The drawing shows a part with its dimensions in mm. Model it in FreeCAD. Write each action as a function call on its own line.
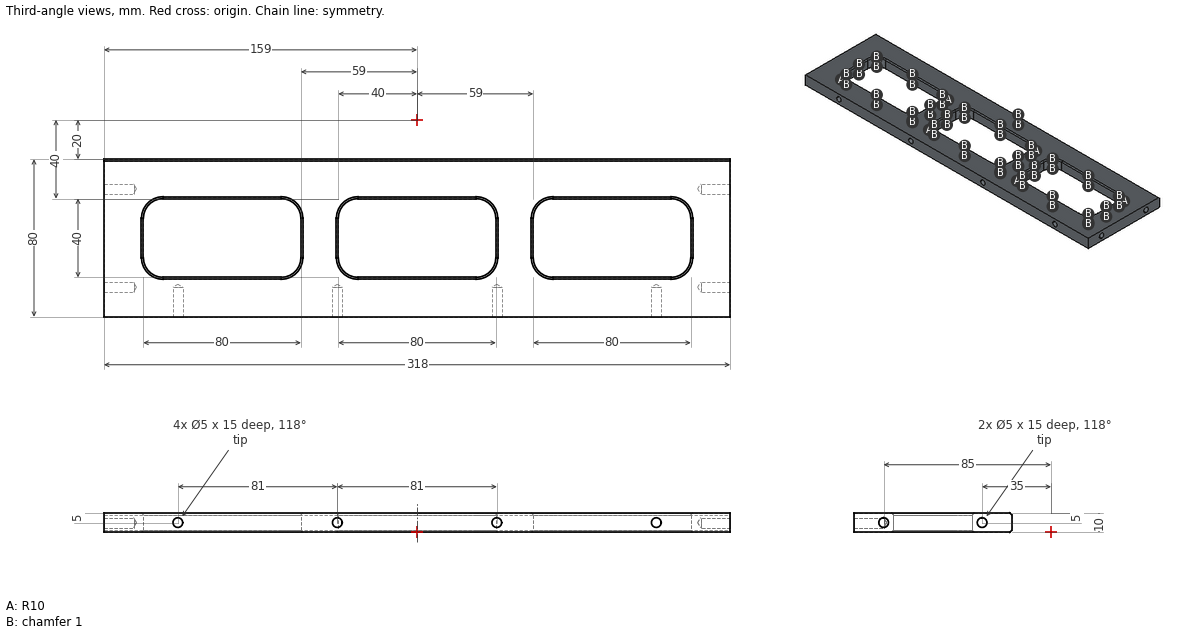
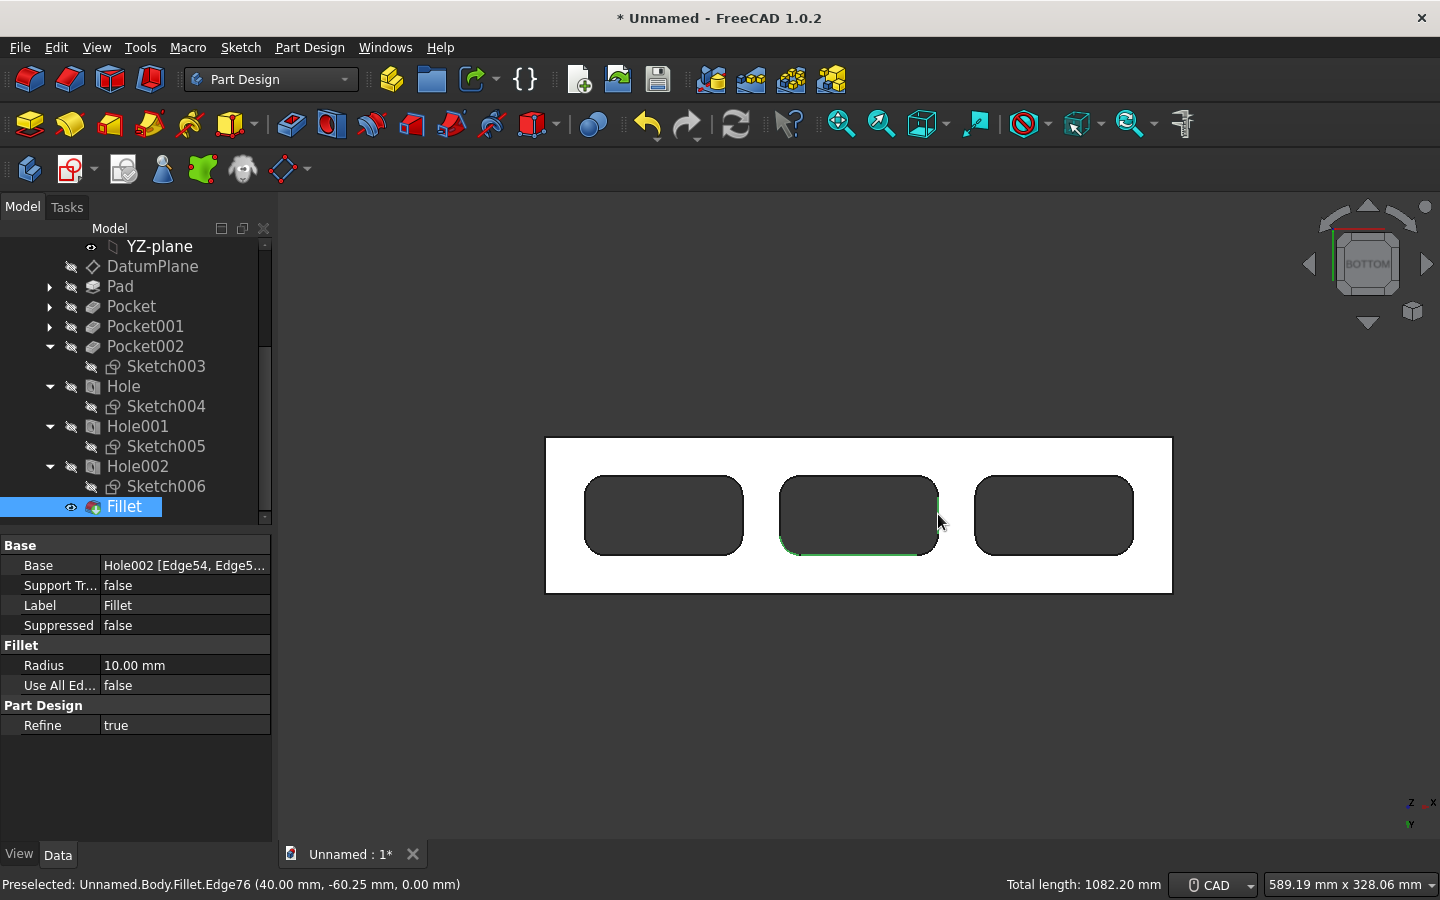
click(1054, 554, ctrl)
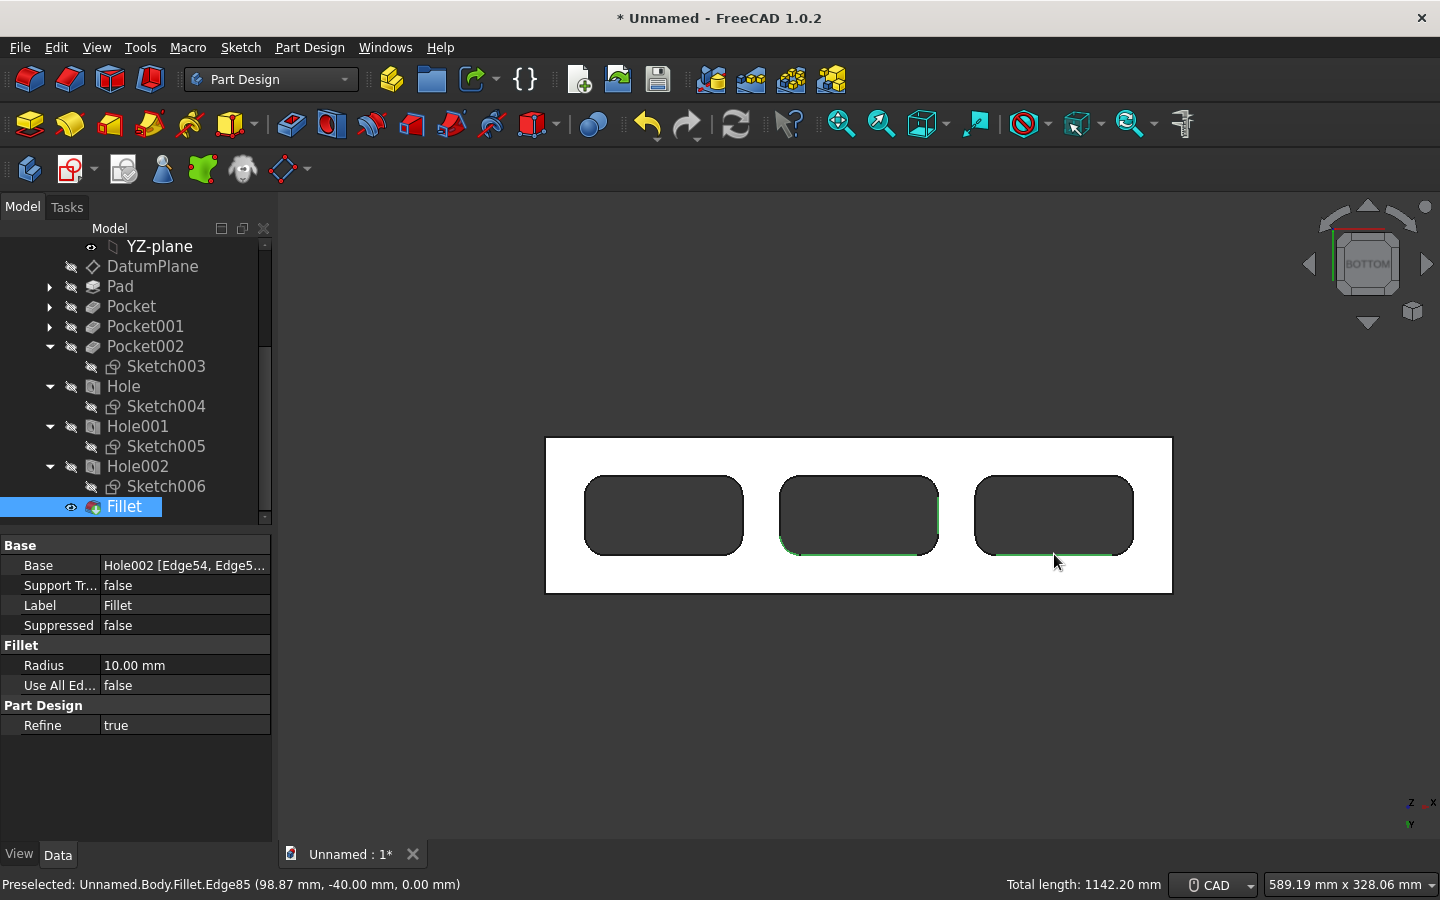
click(1133, 514, ctrl)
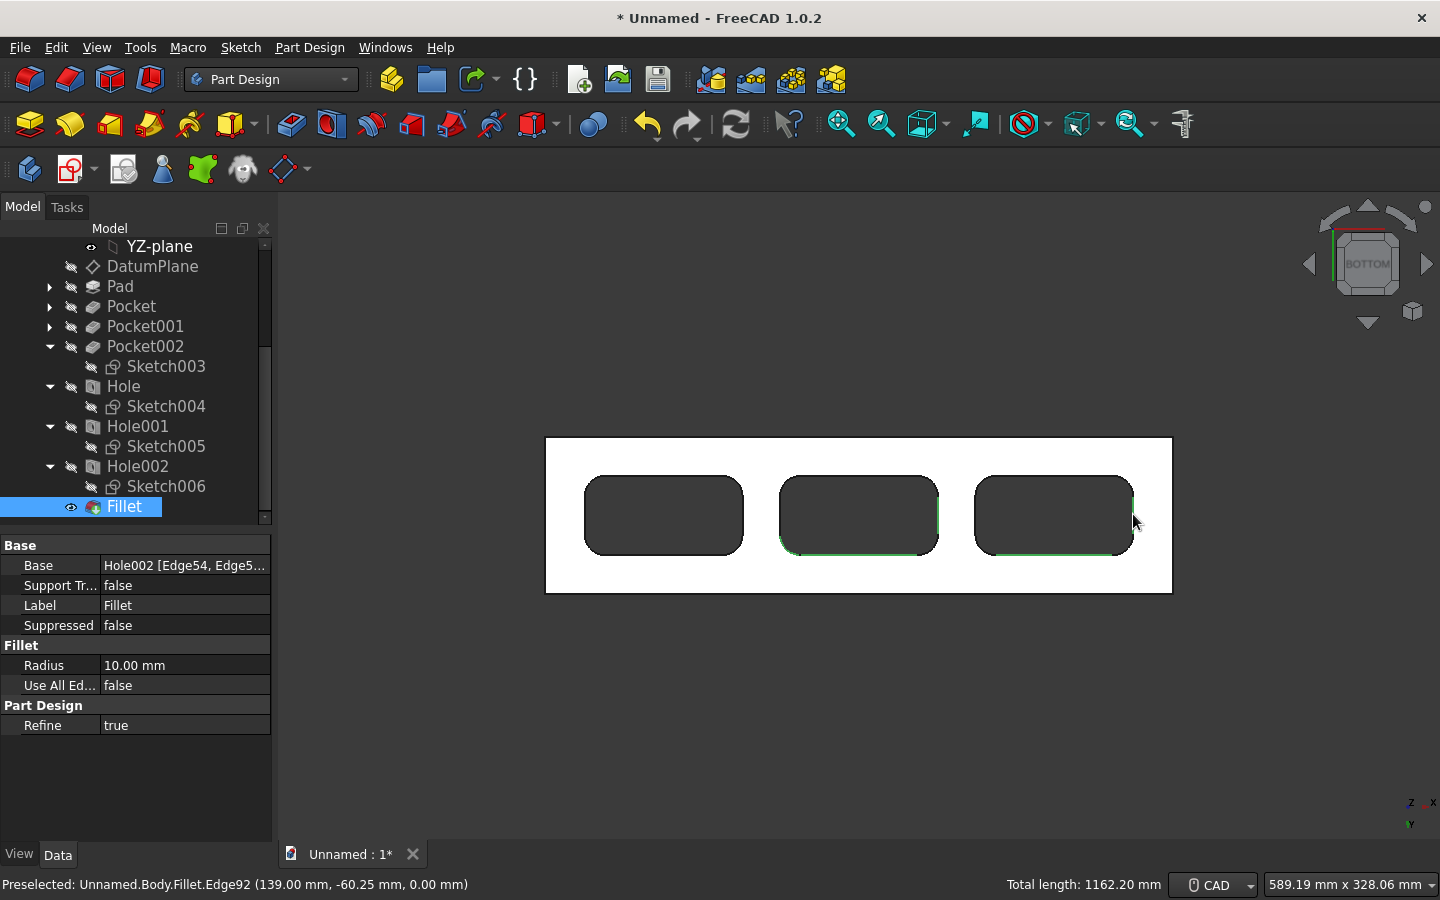
click(859, 475, ctrl)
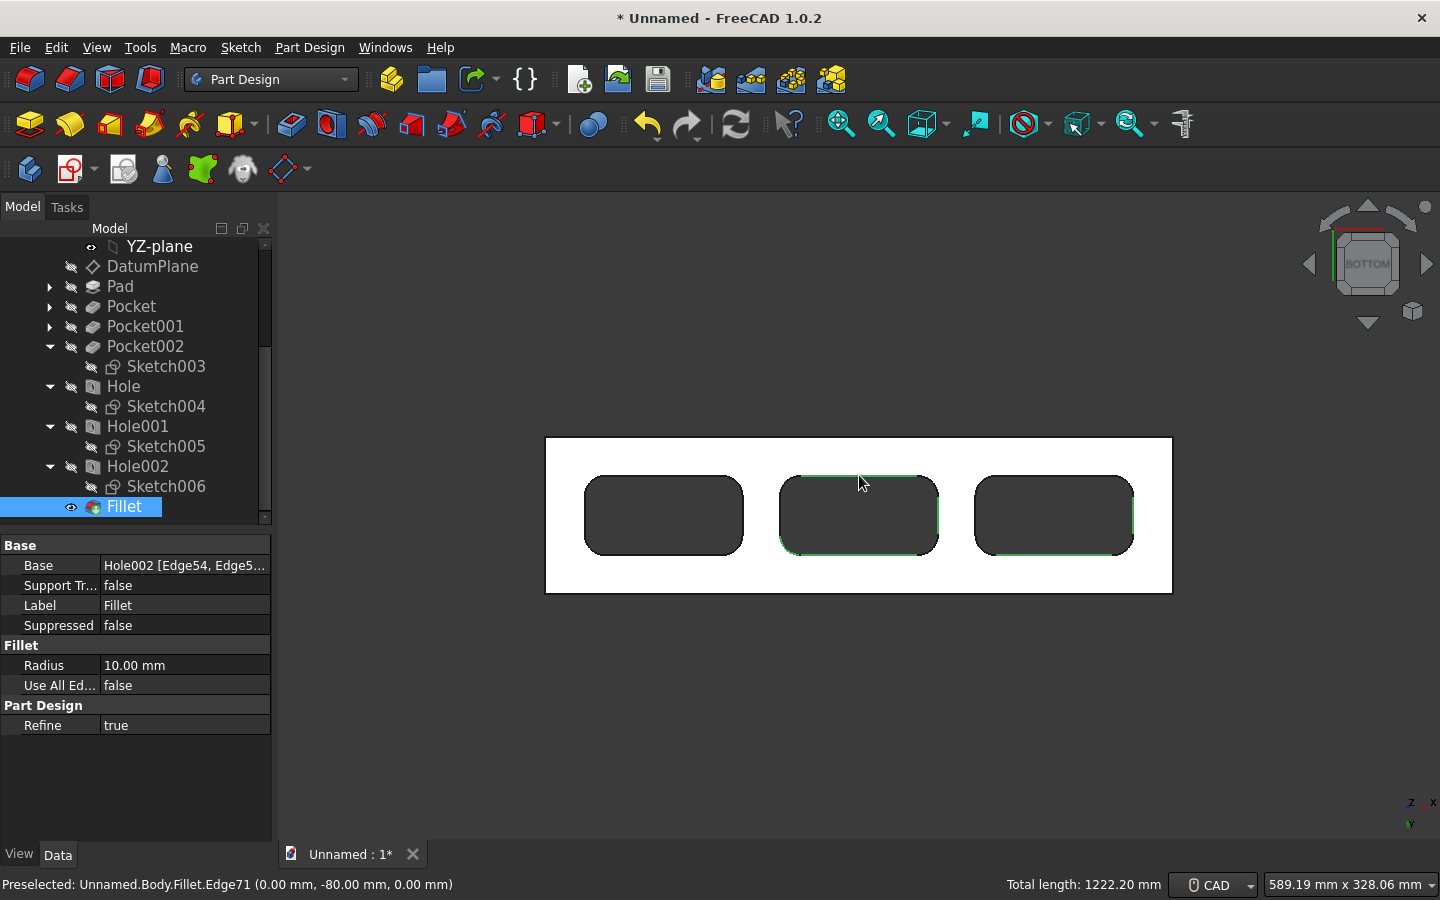
click(780, 514, ctrl)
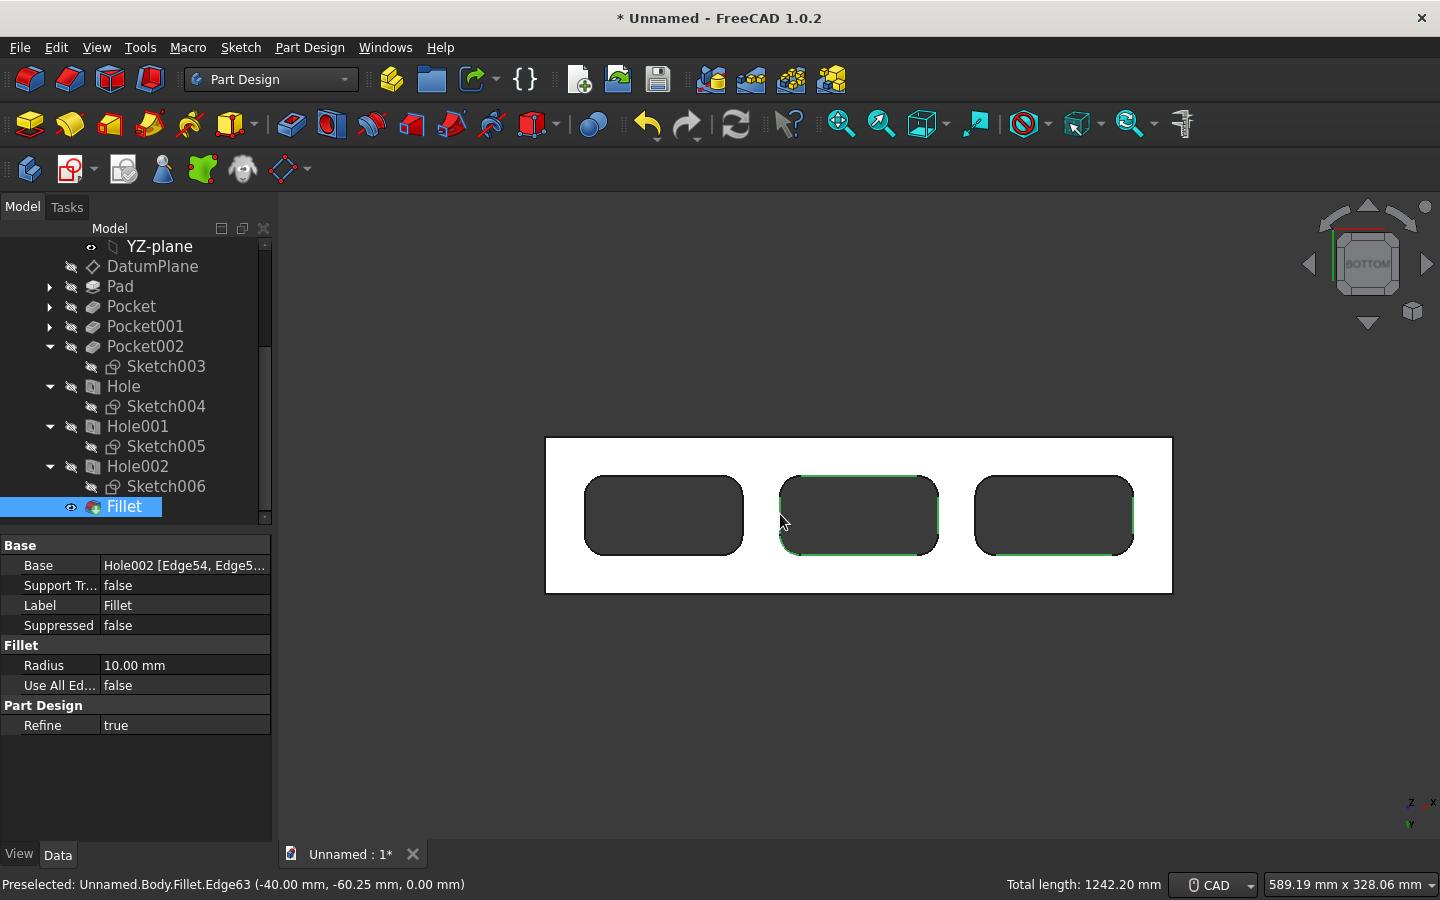
click(1054, 475, ctrl)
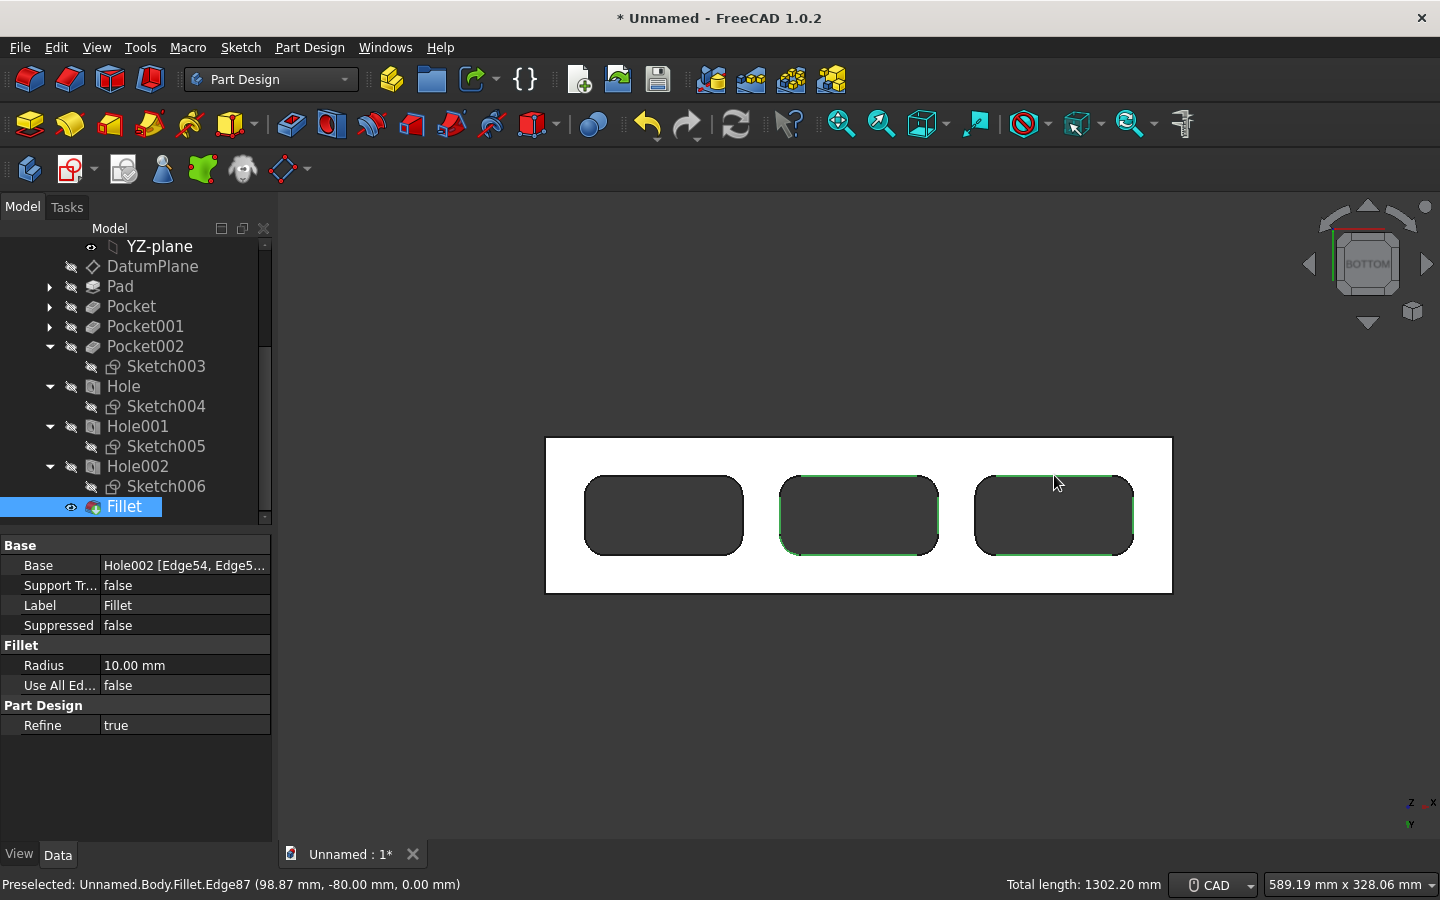
click(664, 554, ctrl)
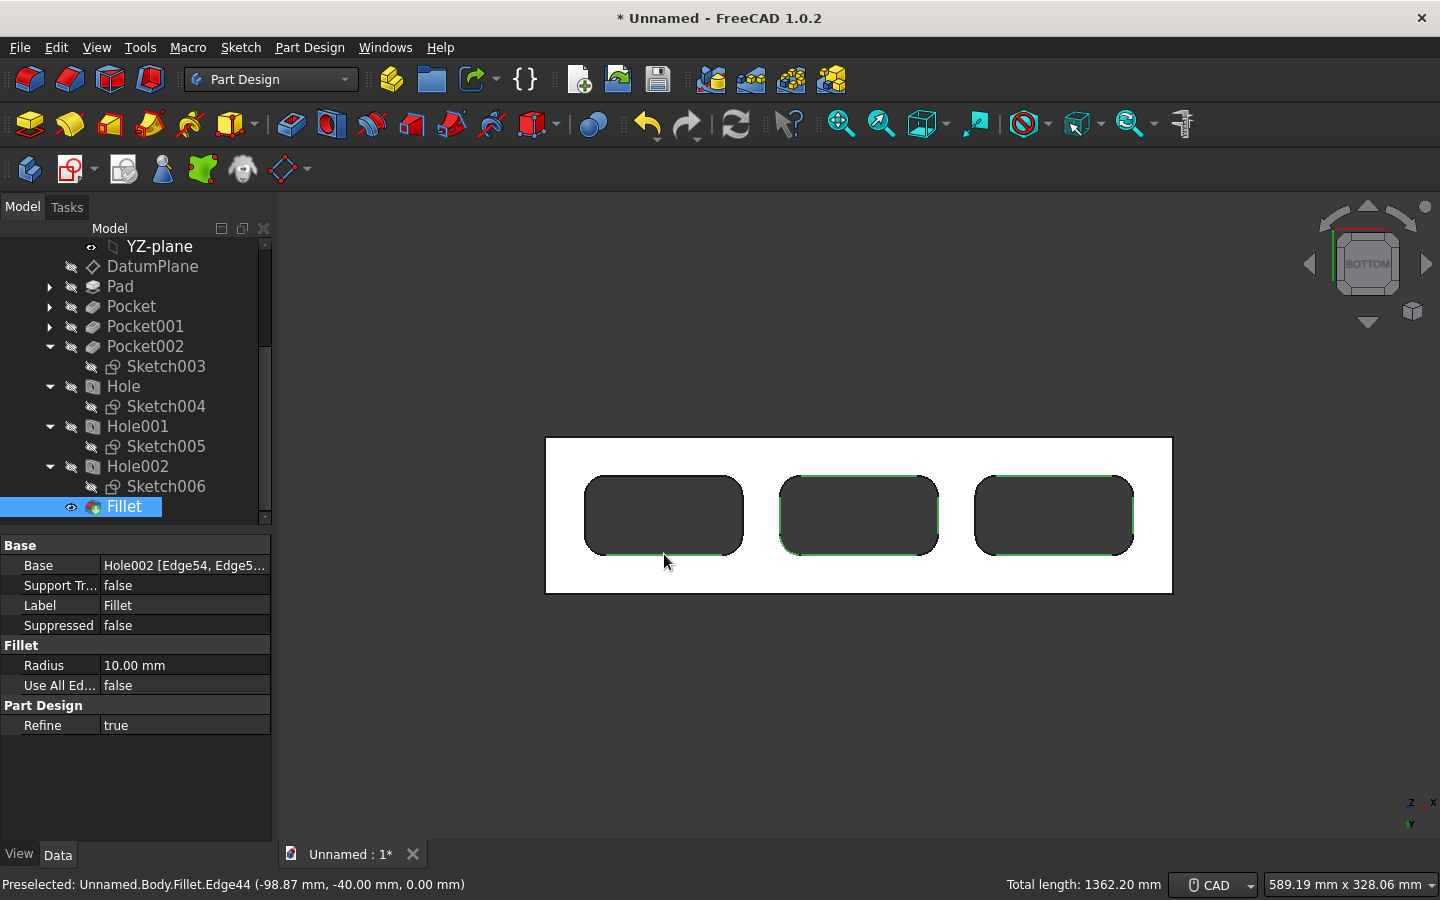
click(585, 514, ctrl)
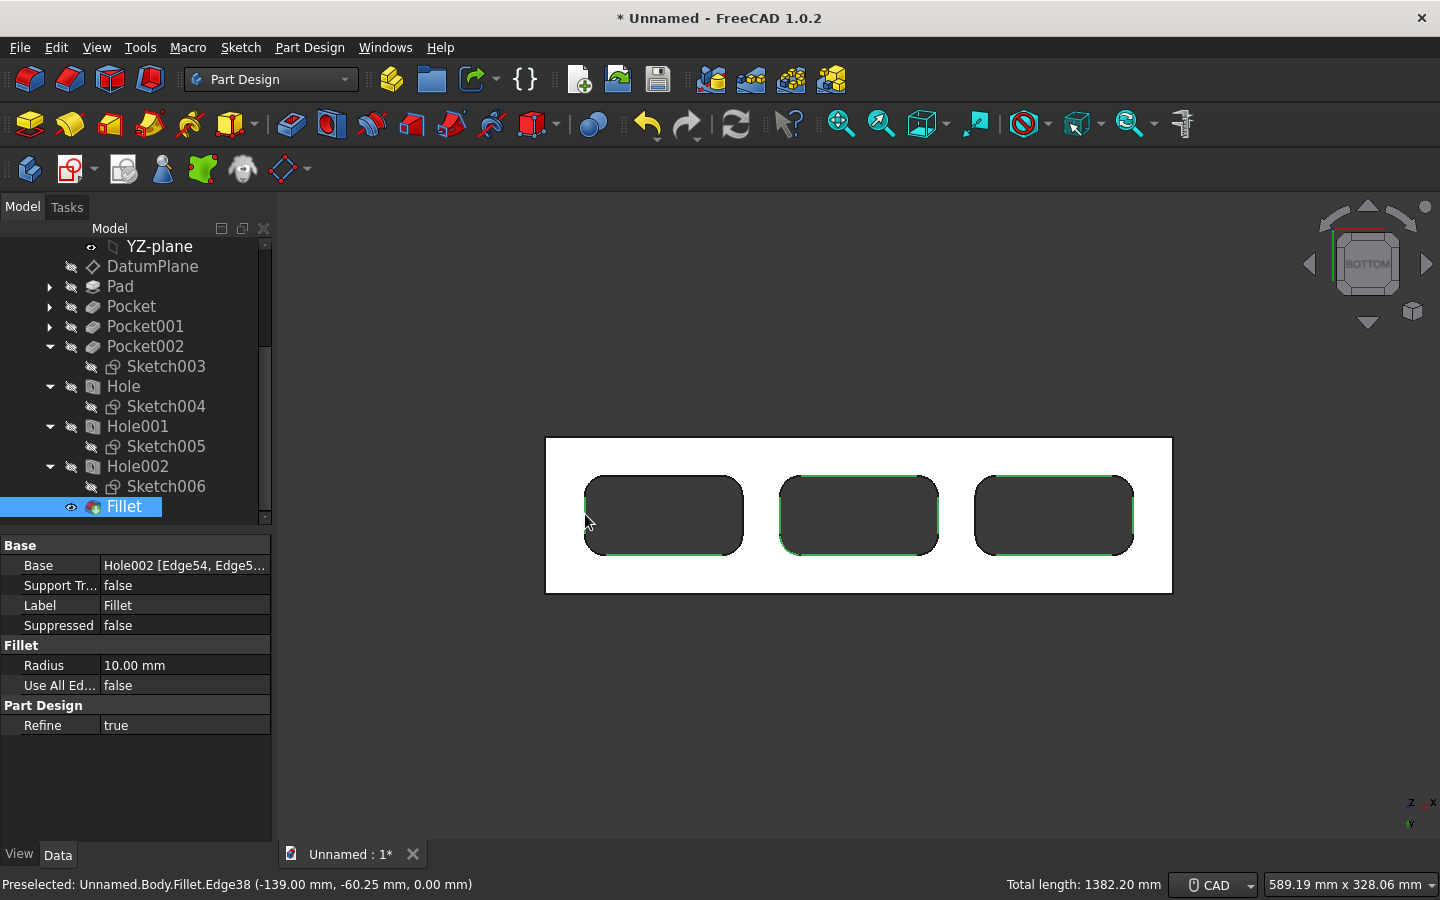
click(975, 514, ctrl)